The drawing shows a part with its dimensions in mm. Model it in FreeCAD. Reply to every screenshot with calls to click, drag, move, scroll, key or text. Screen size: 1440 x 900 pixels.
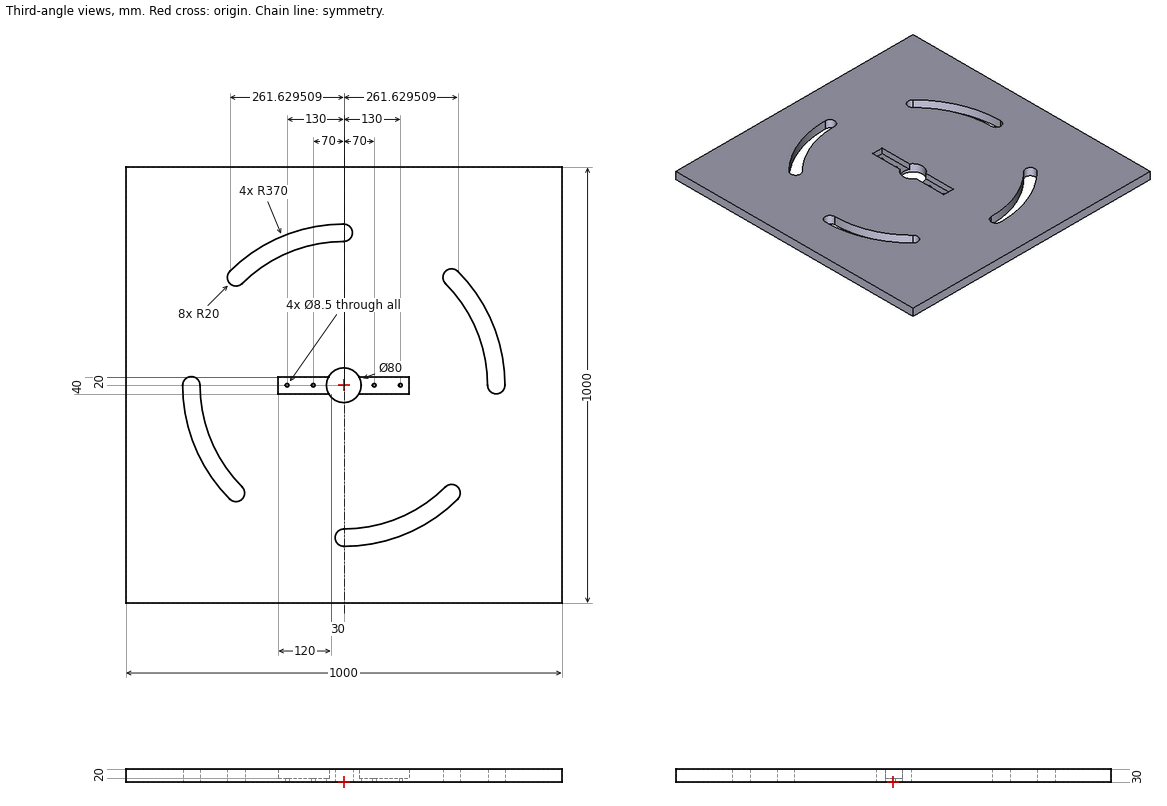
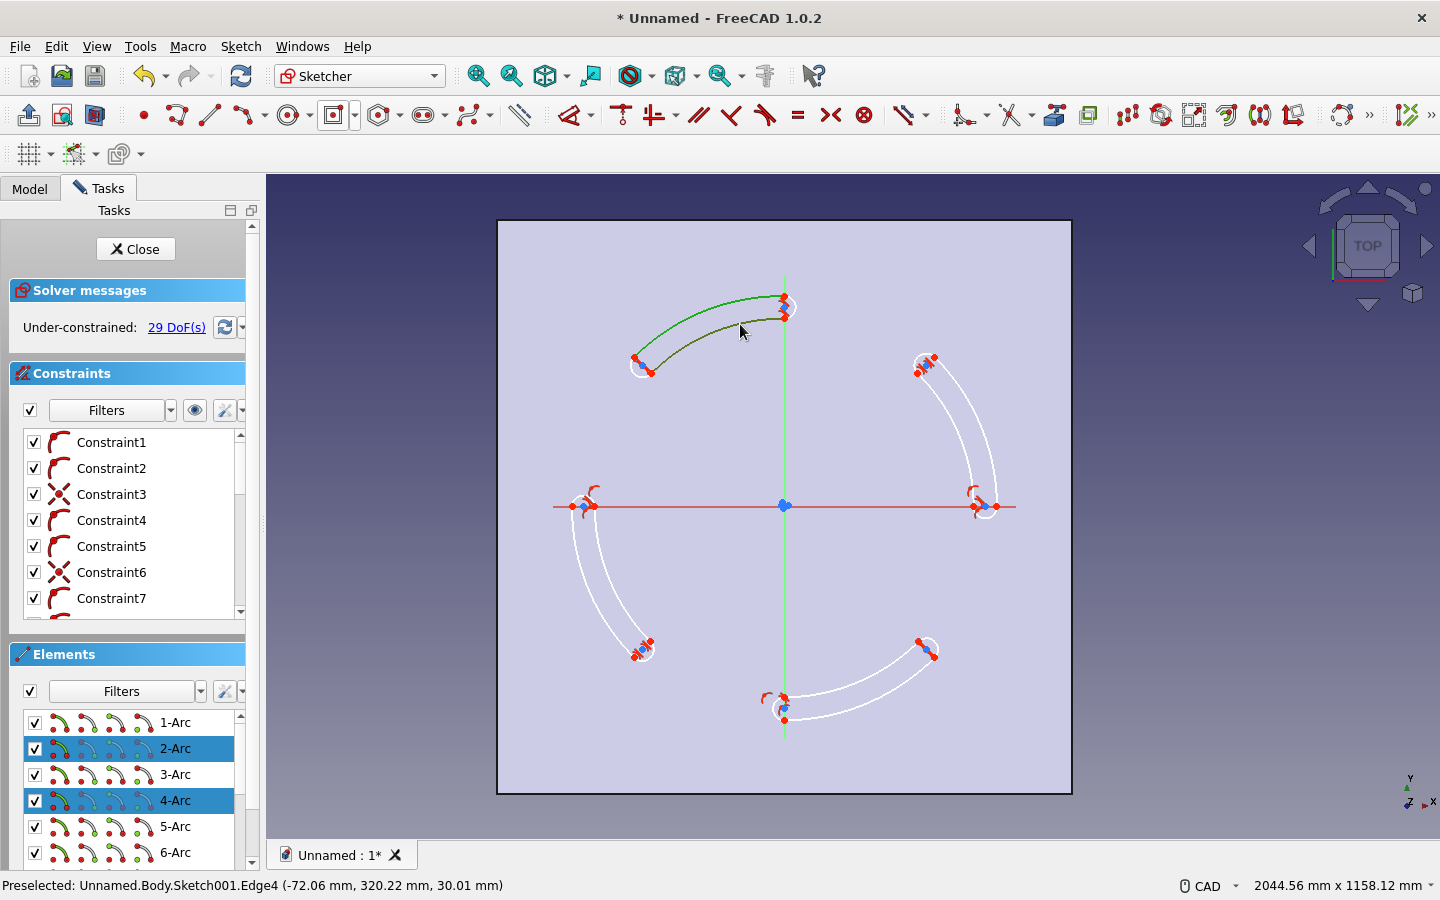
click(621, 116)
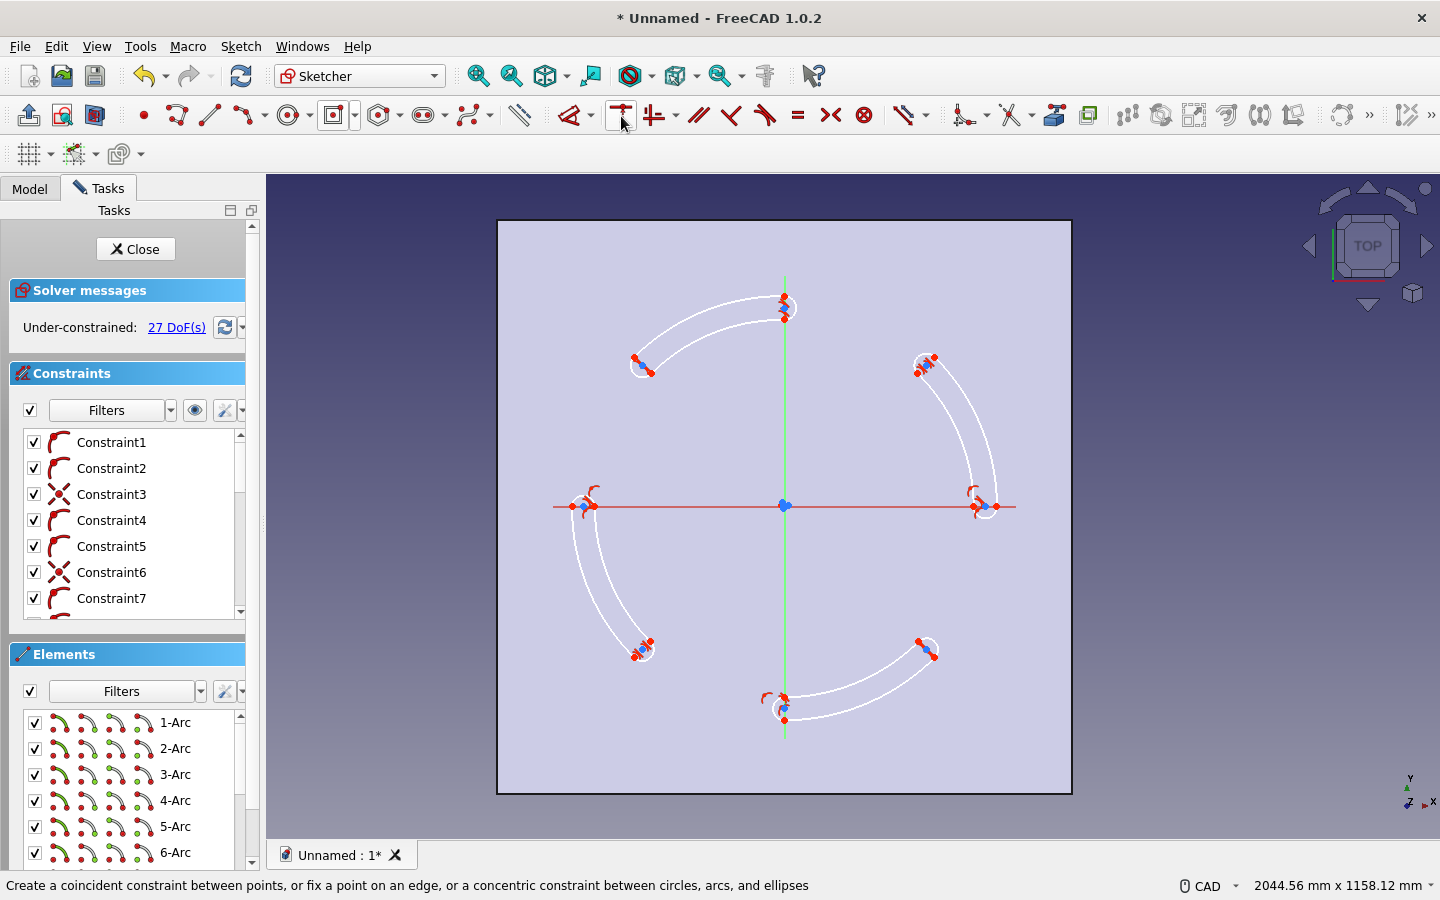
click(735, 301)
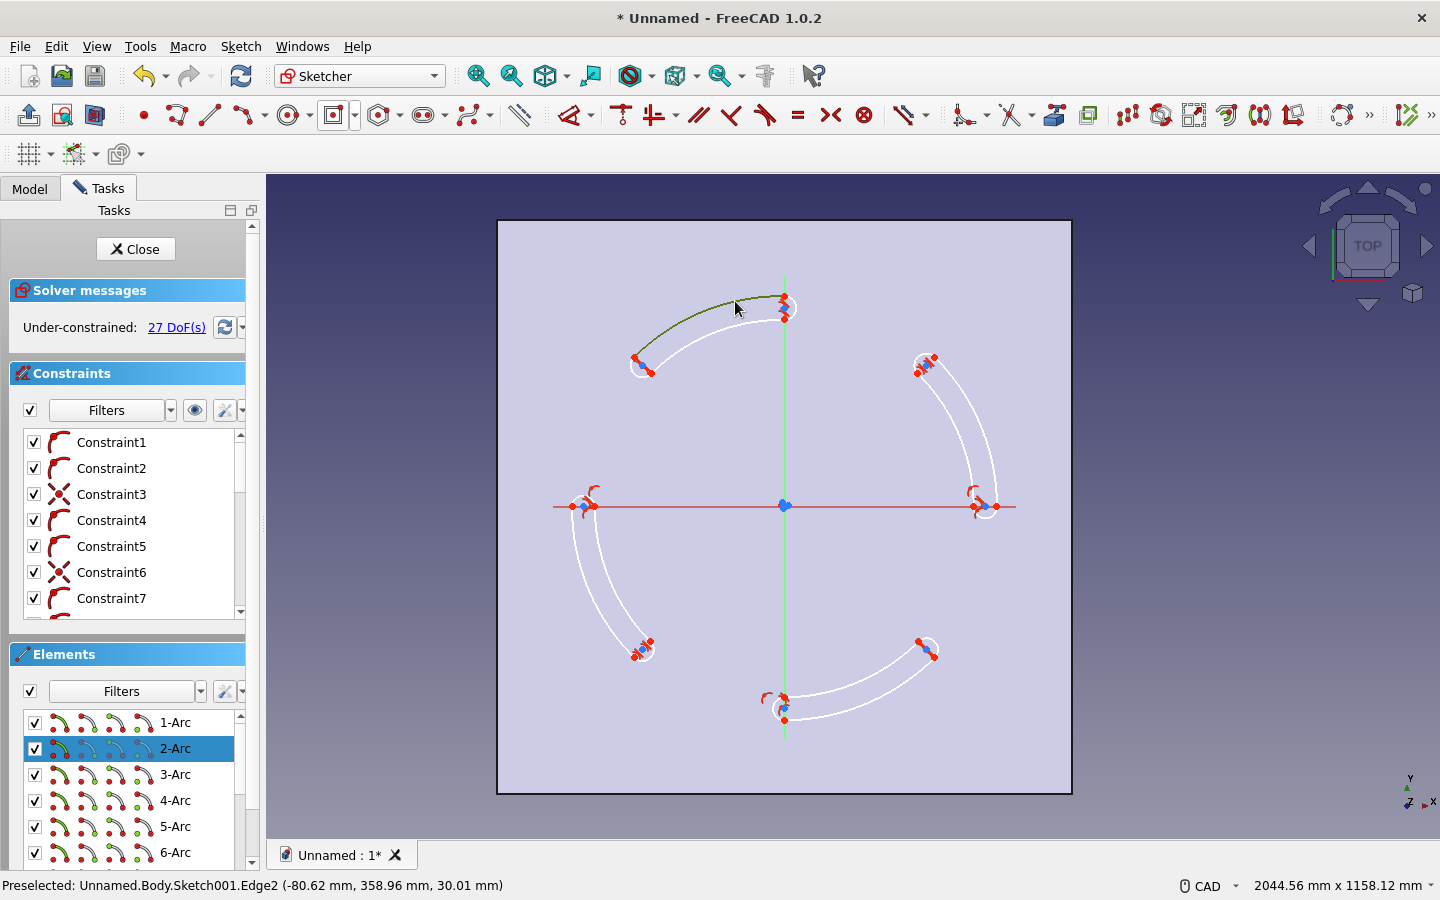
click(991, 457)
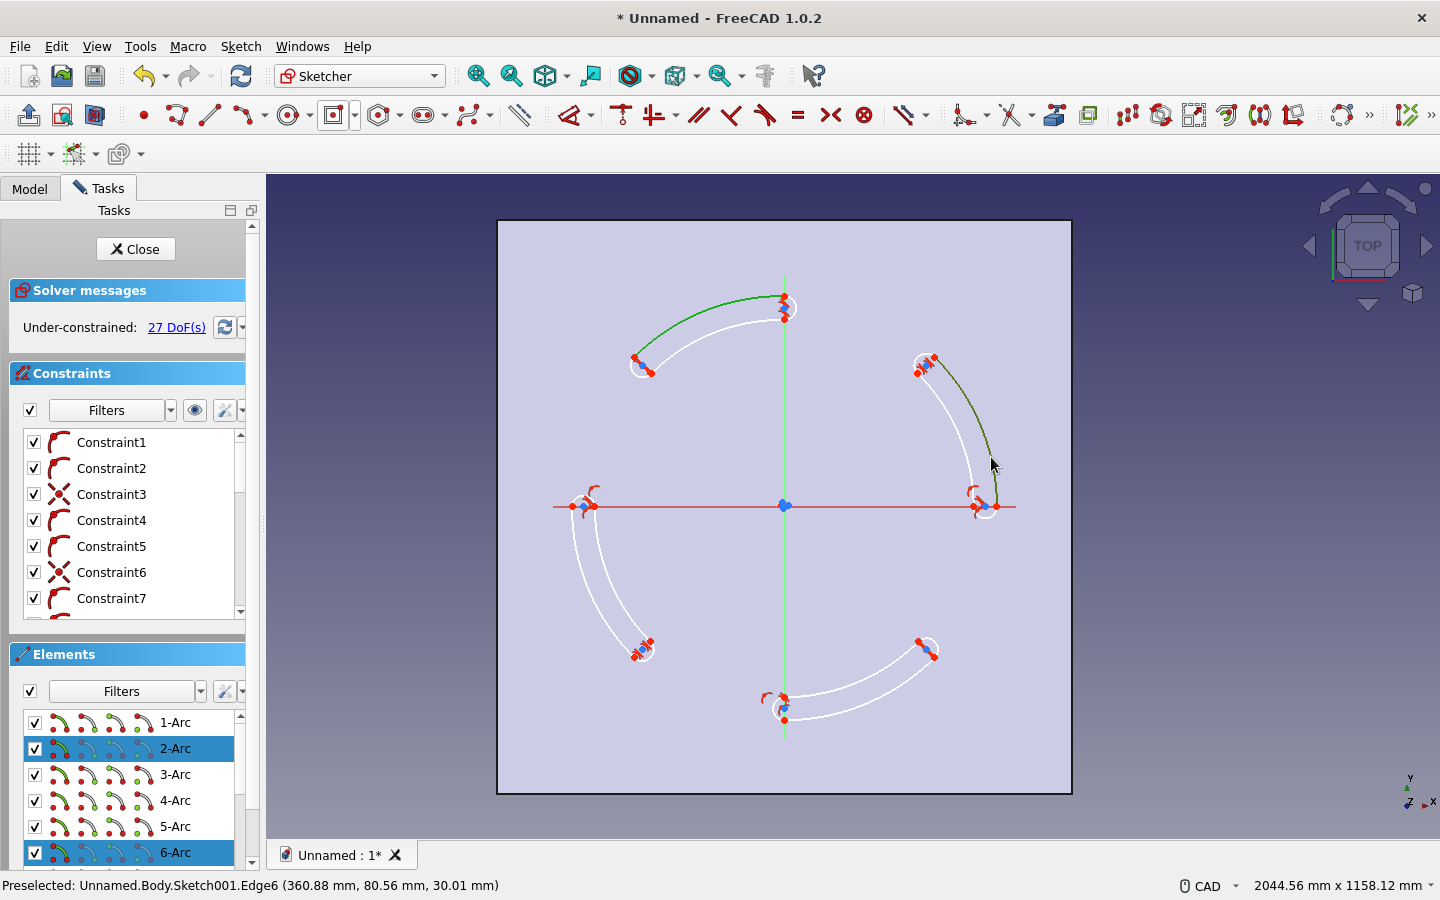
click(621, 116)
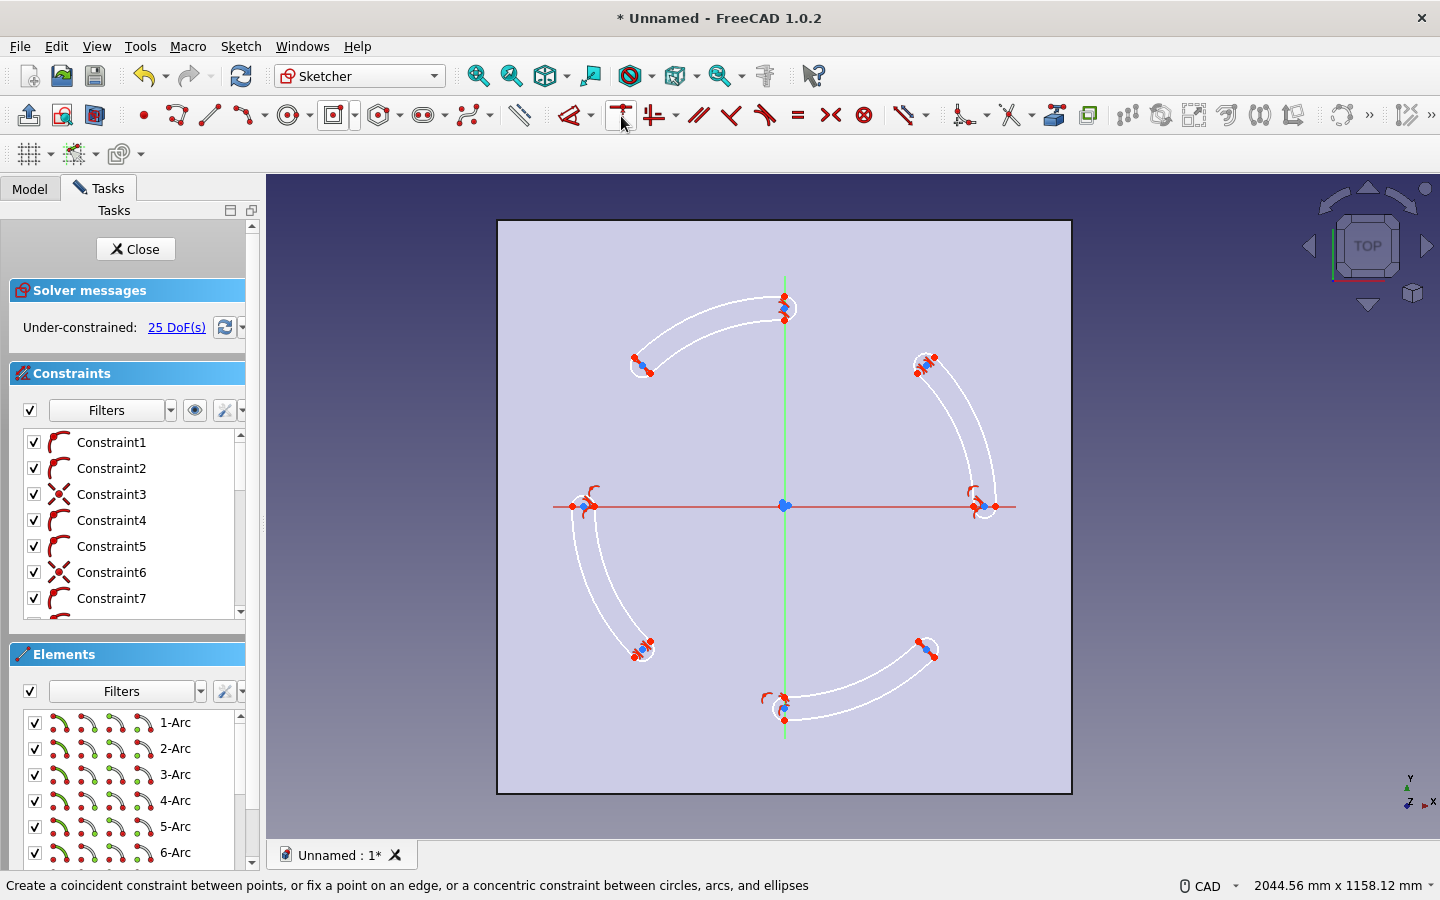
click(735, 302)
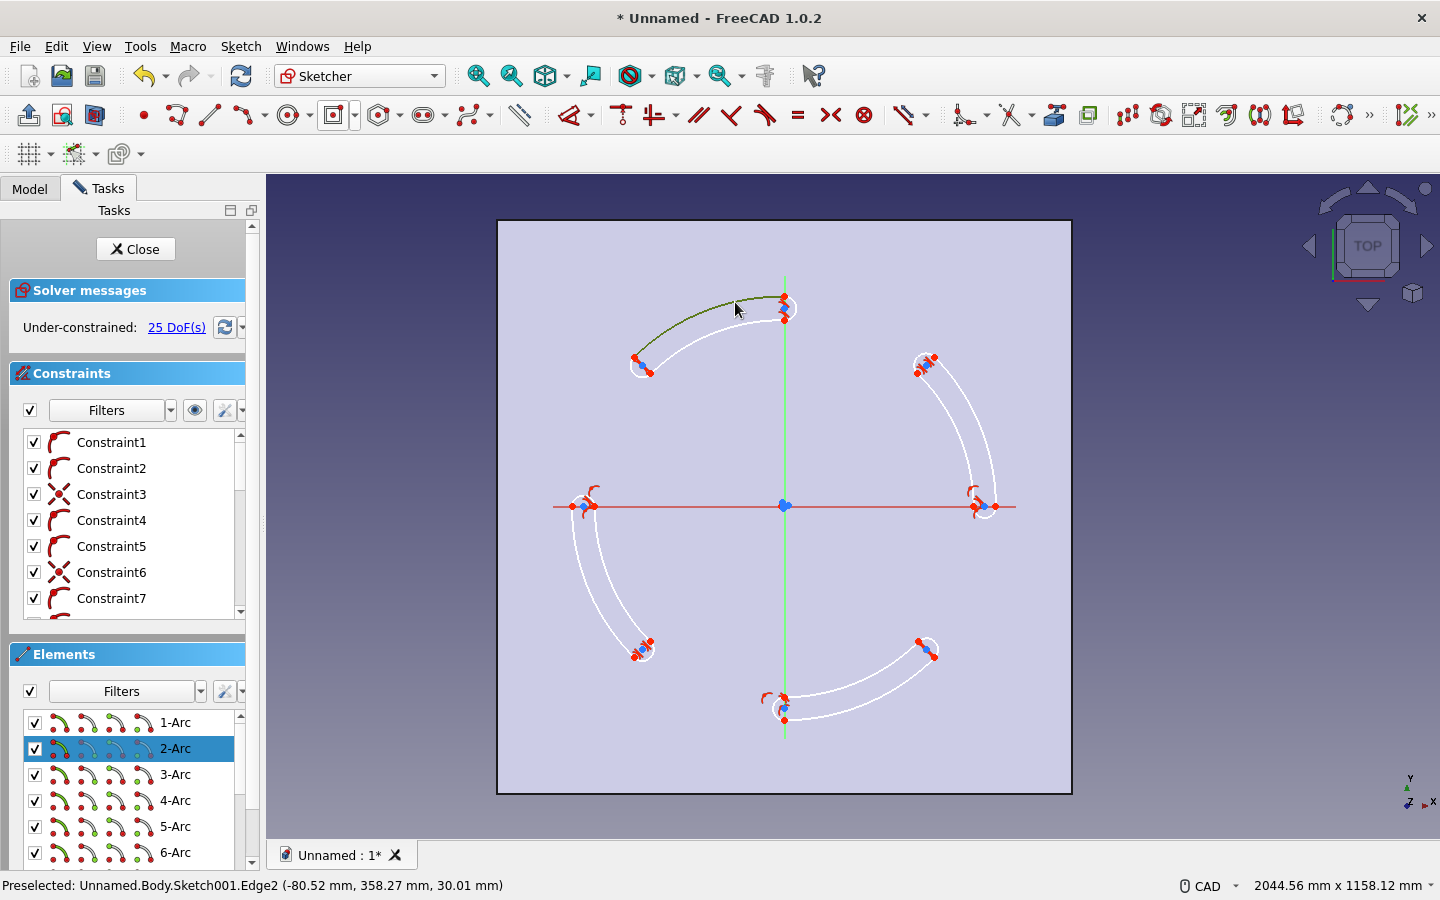
click(968, 463)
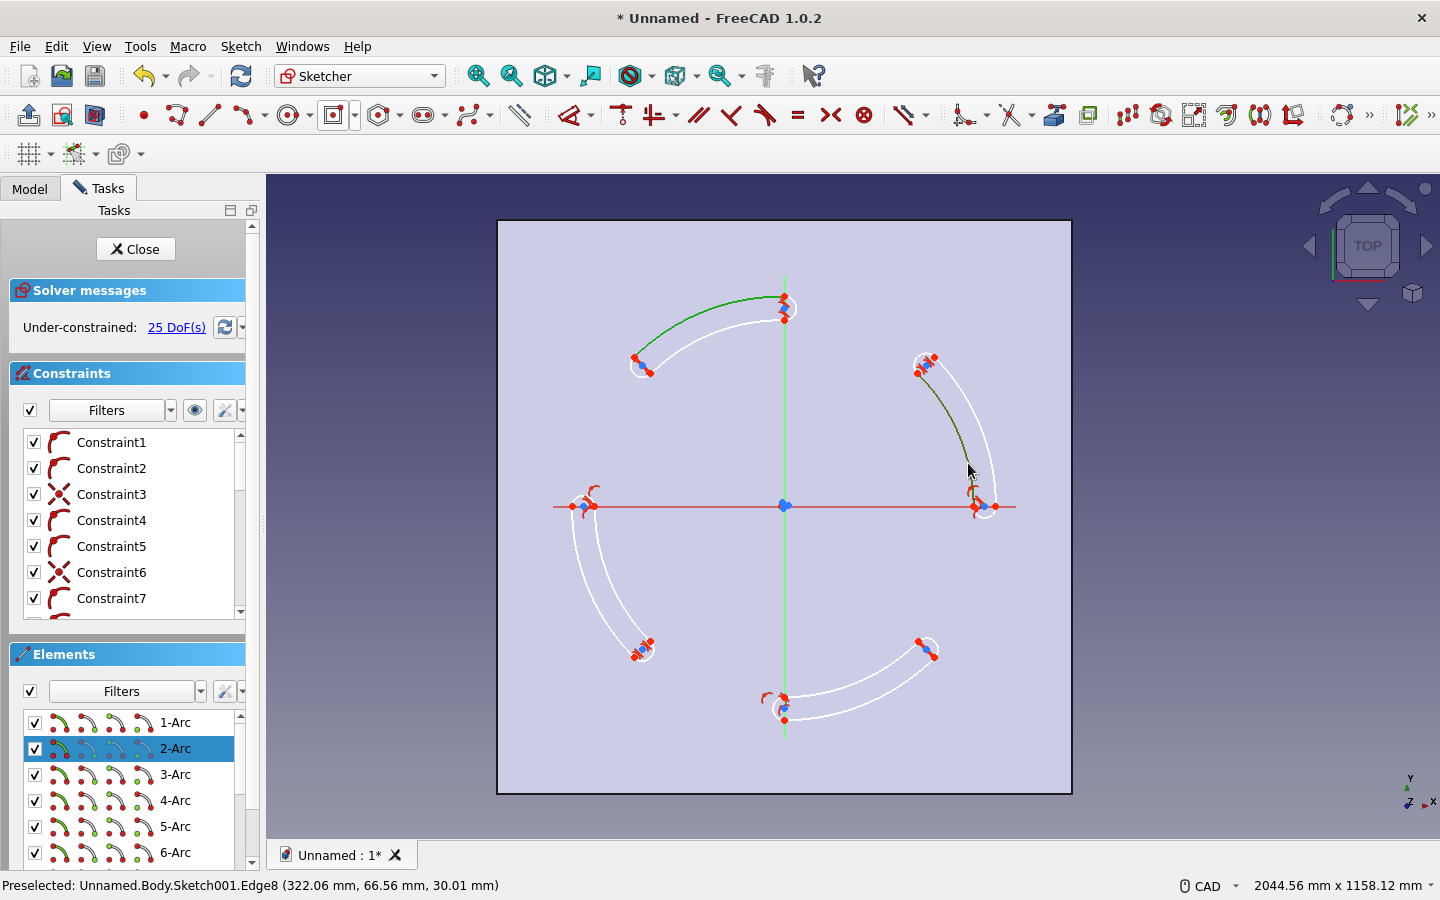
key(c)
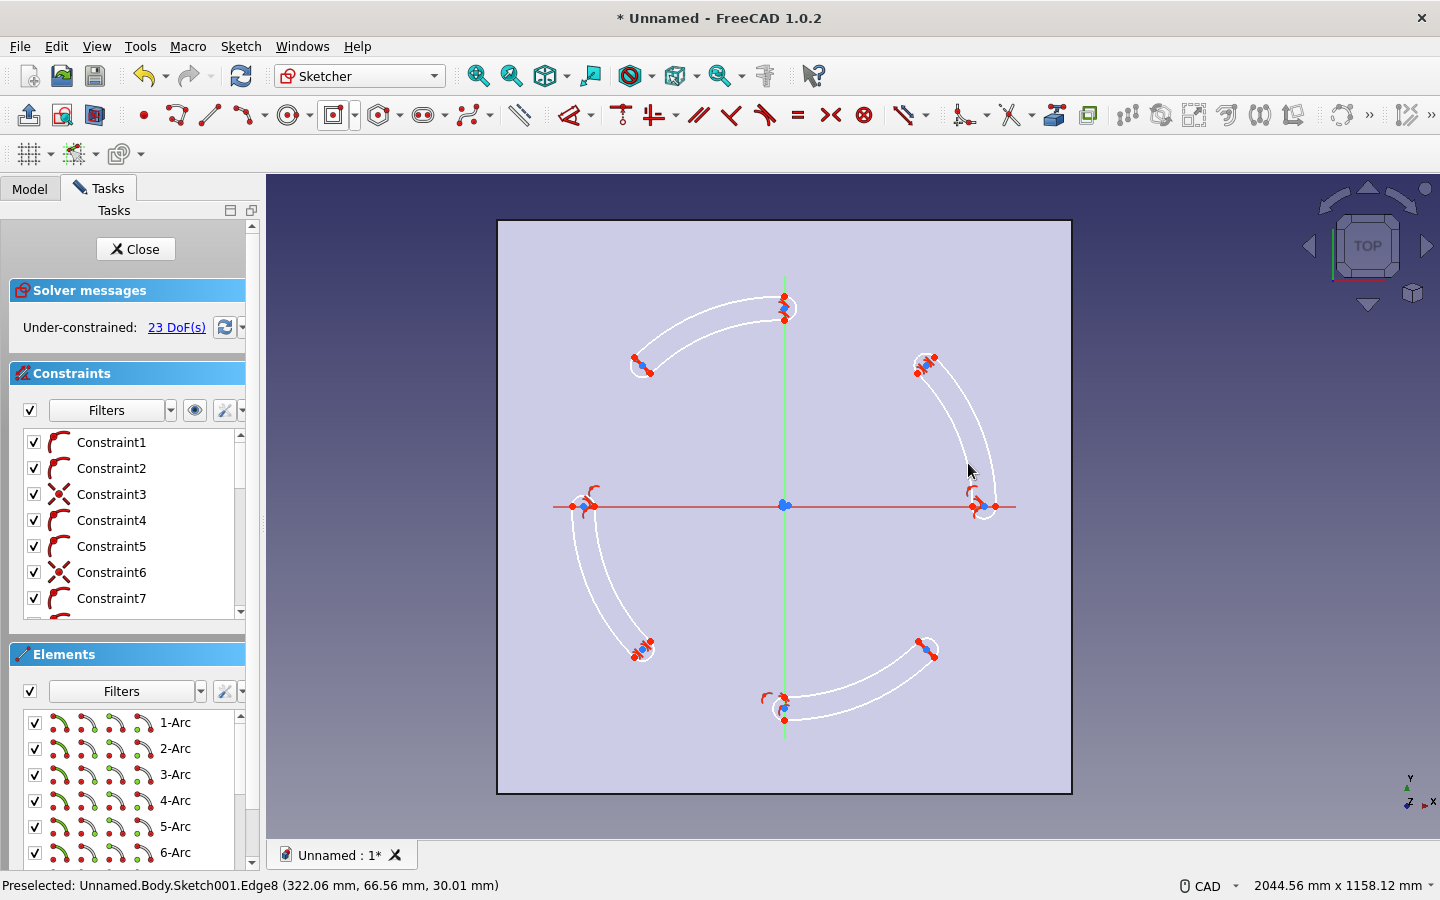
click(735, 302)